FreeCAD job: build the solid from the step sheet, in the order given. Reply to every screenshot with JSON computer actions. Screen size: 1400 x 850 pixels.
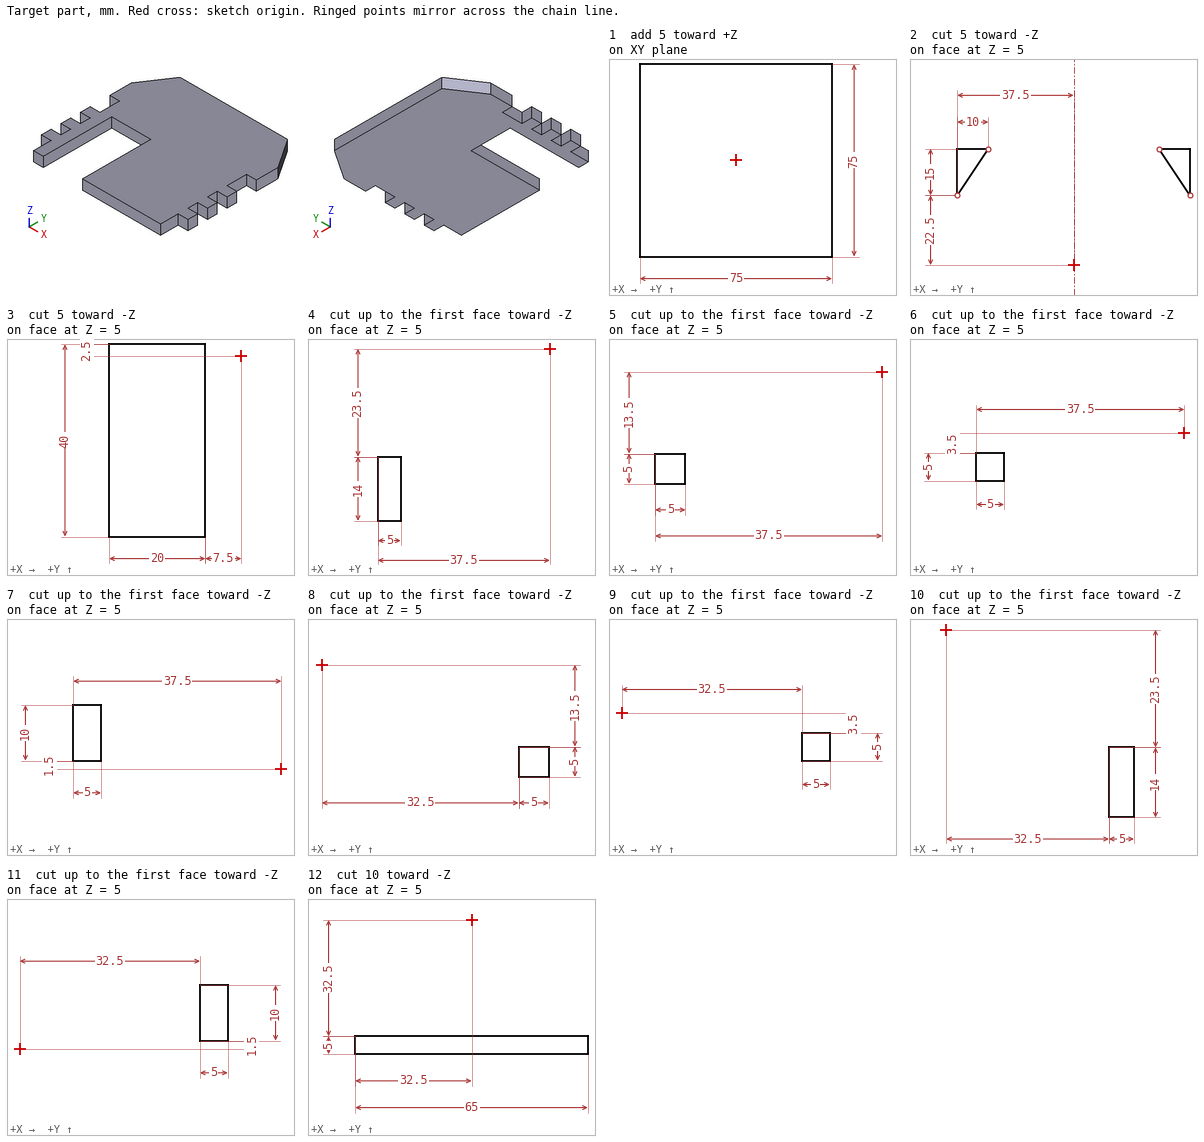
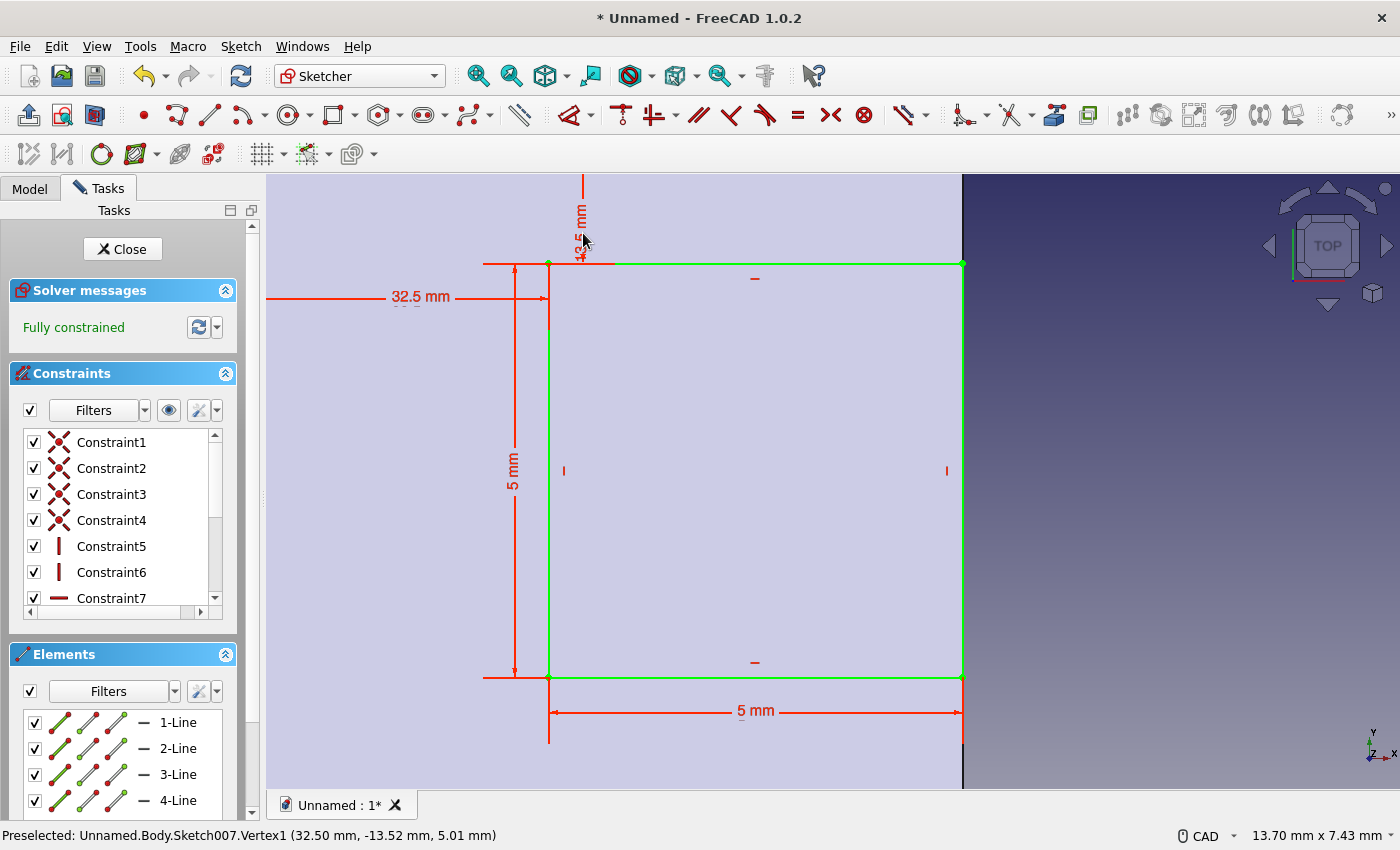
{"action": "left_click", "coordinate": [123, 249]}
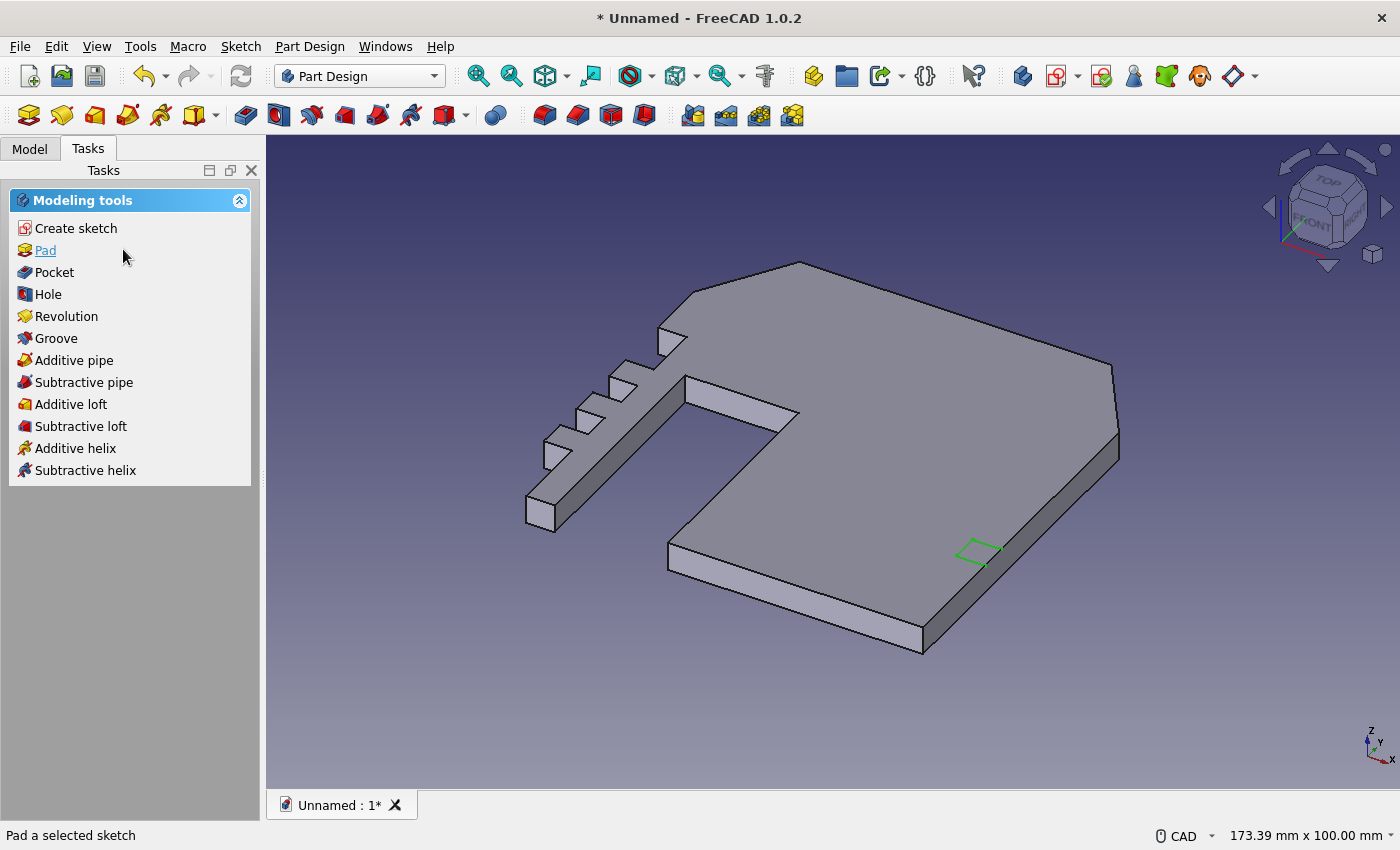
{"action": "left_click", "coordinate": [246, 116]}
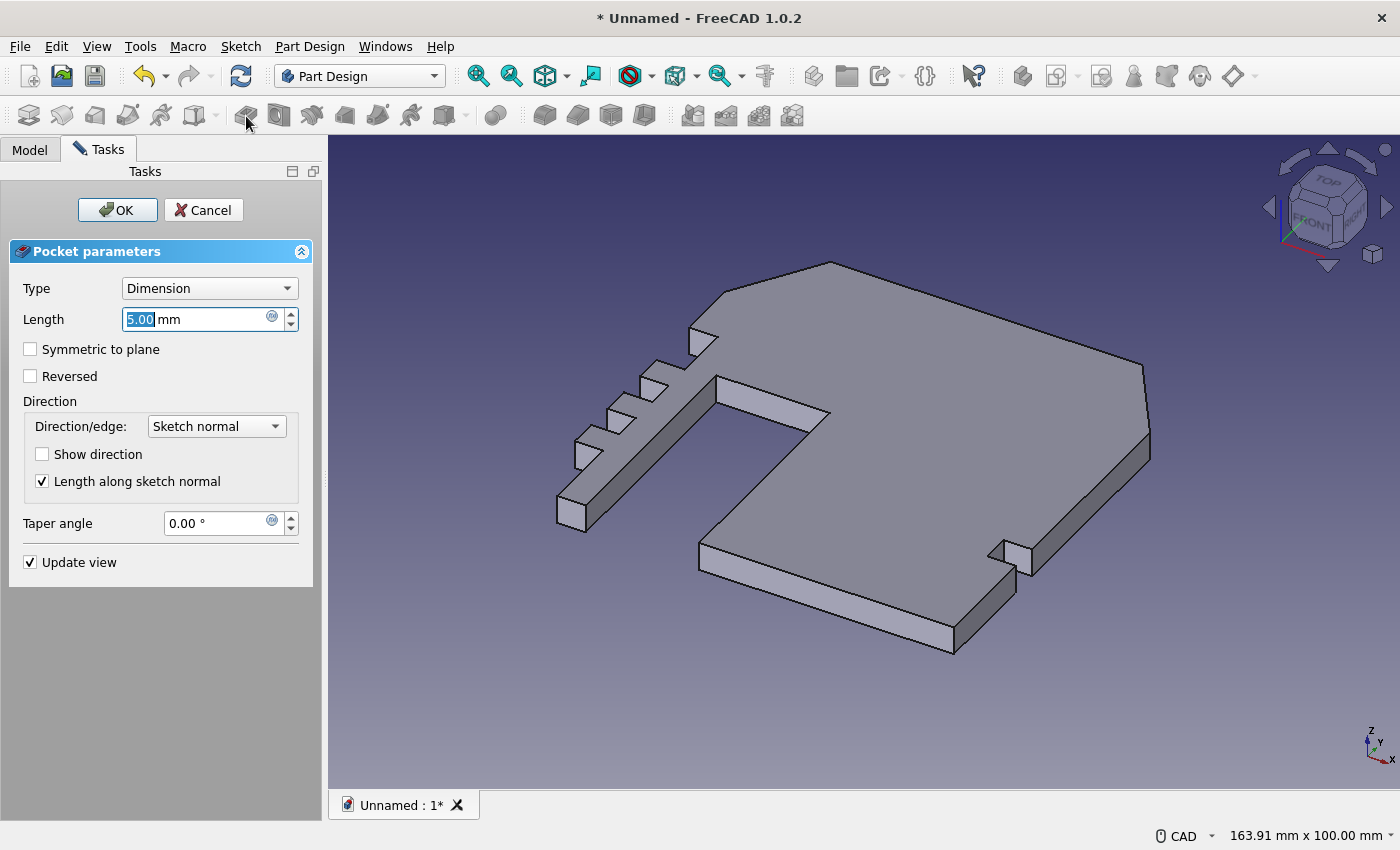
{"action": "left_click", "coordinate": [210, 288]}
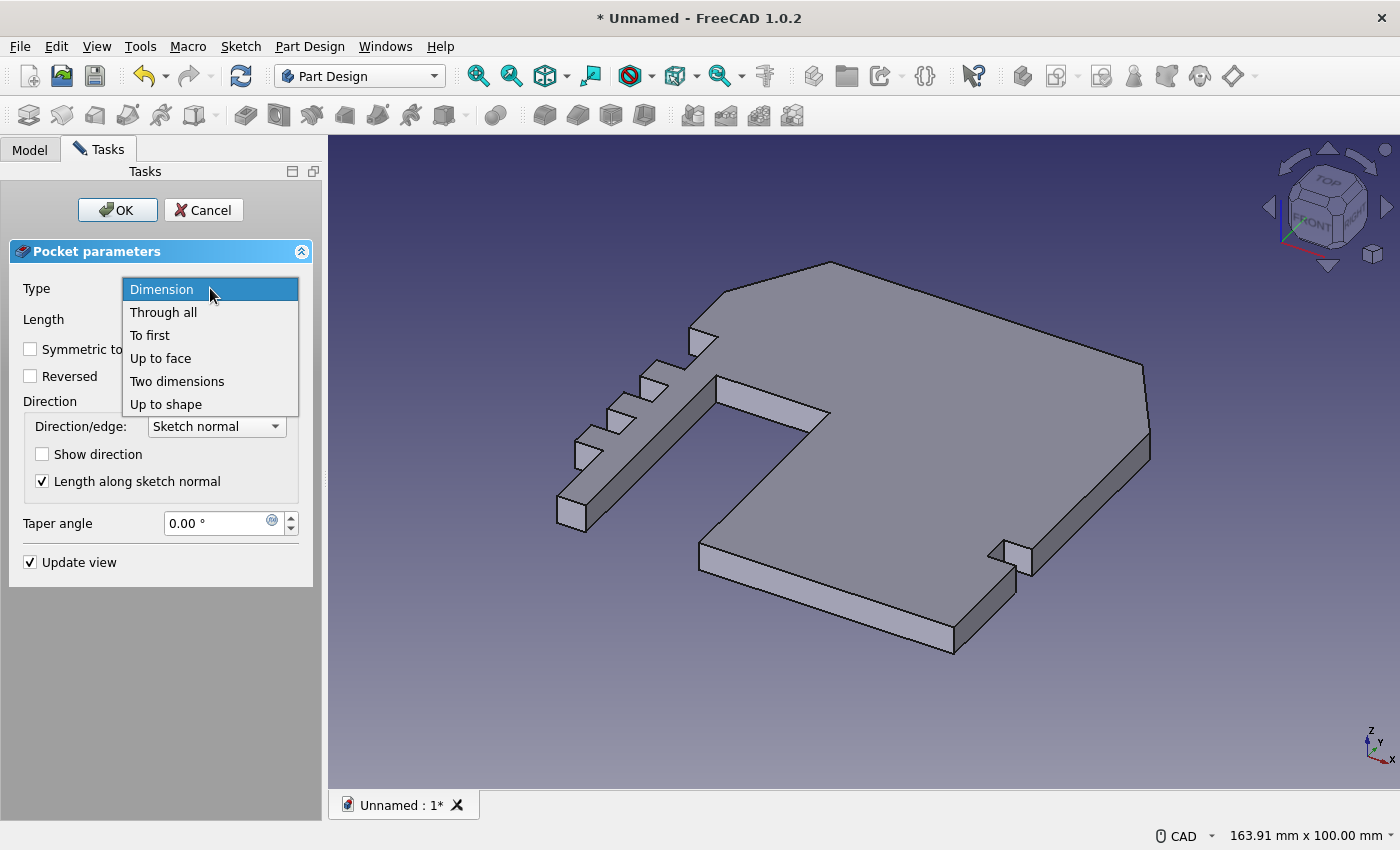
{"action": "left_click", "coordinate": [208, 336]}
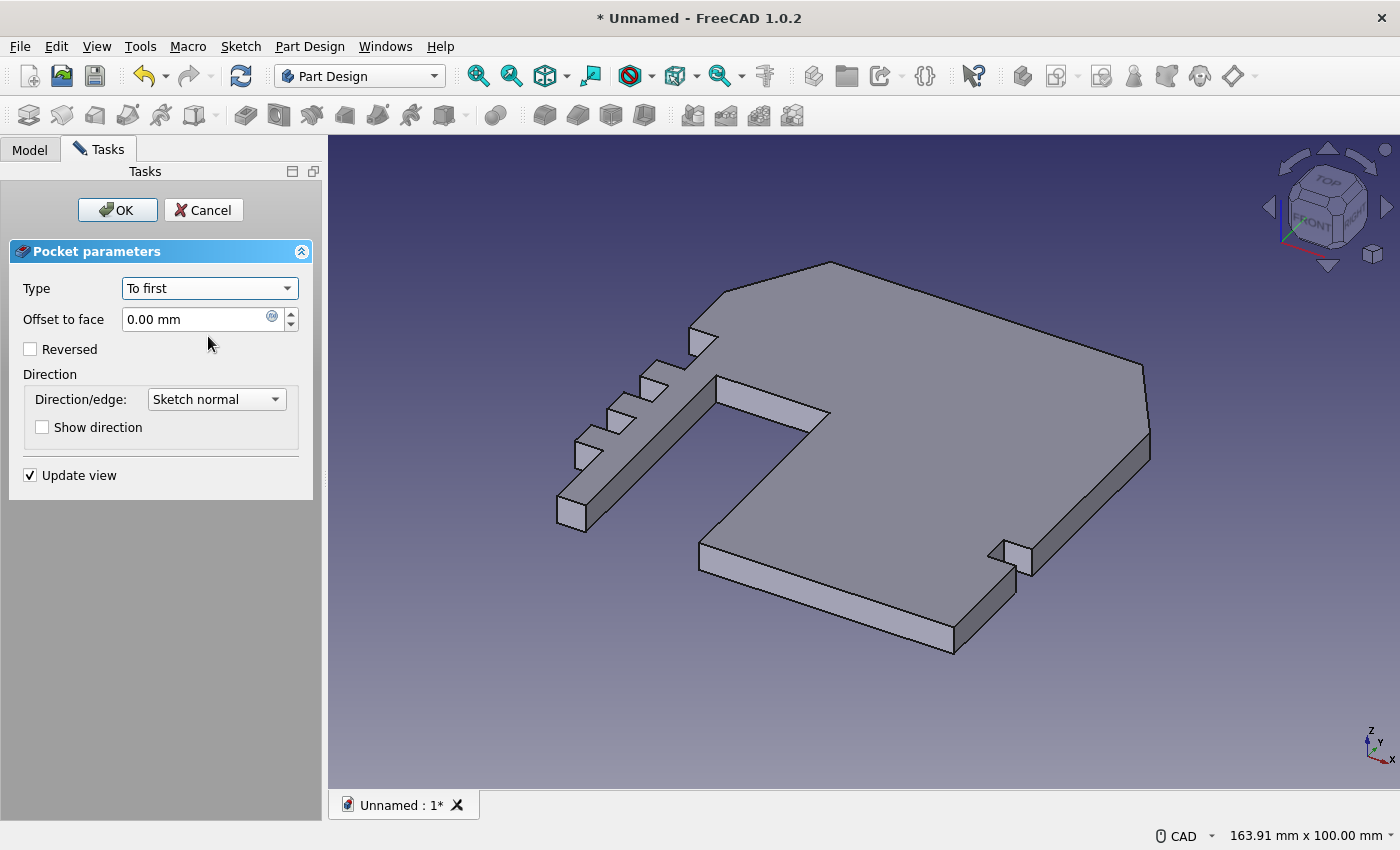
{"action": "left_click", "coordinate": [118, 210]}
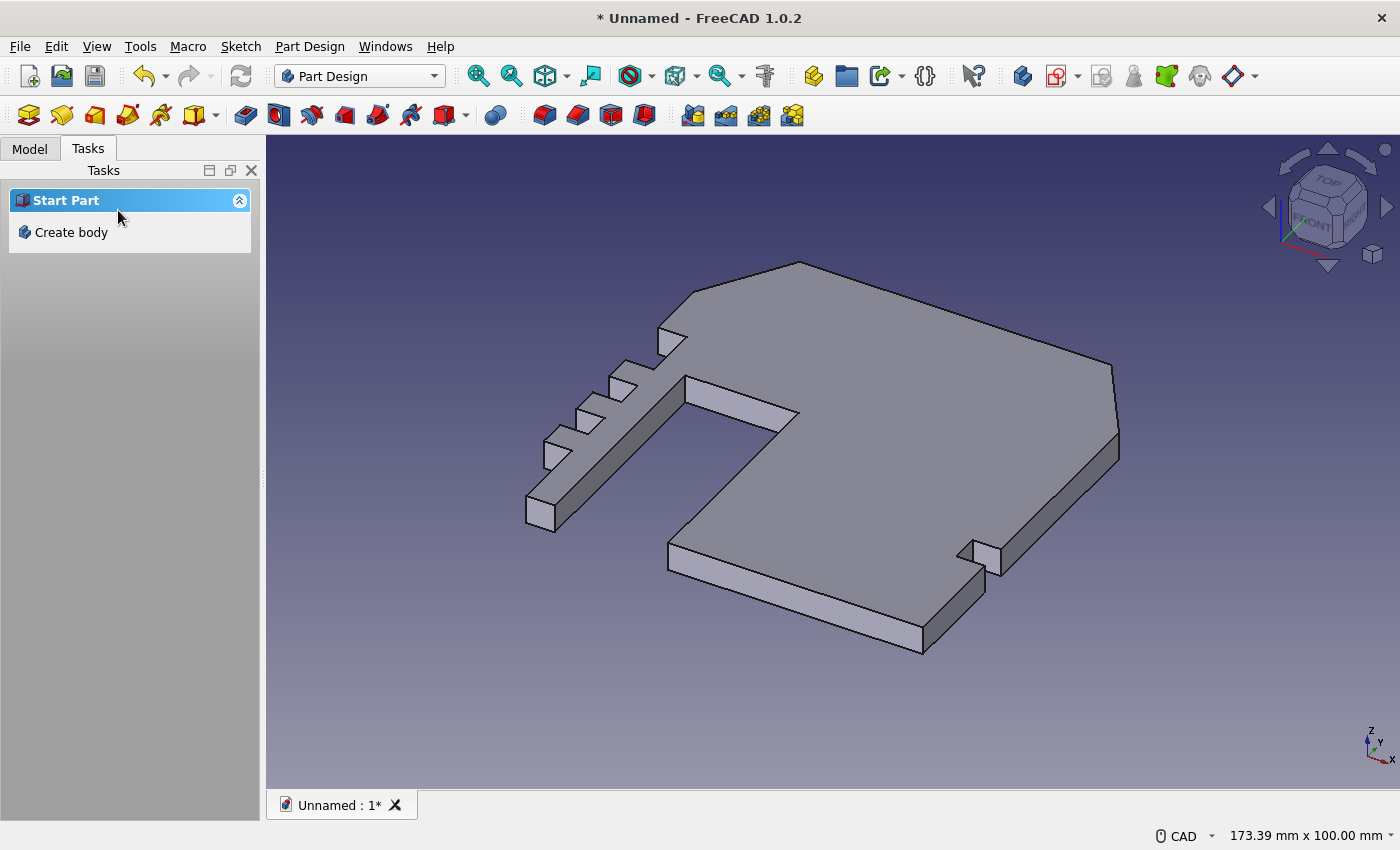
{"action": "left_click", "coordinate": [929, 420]}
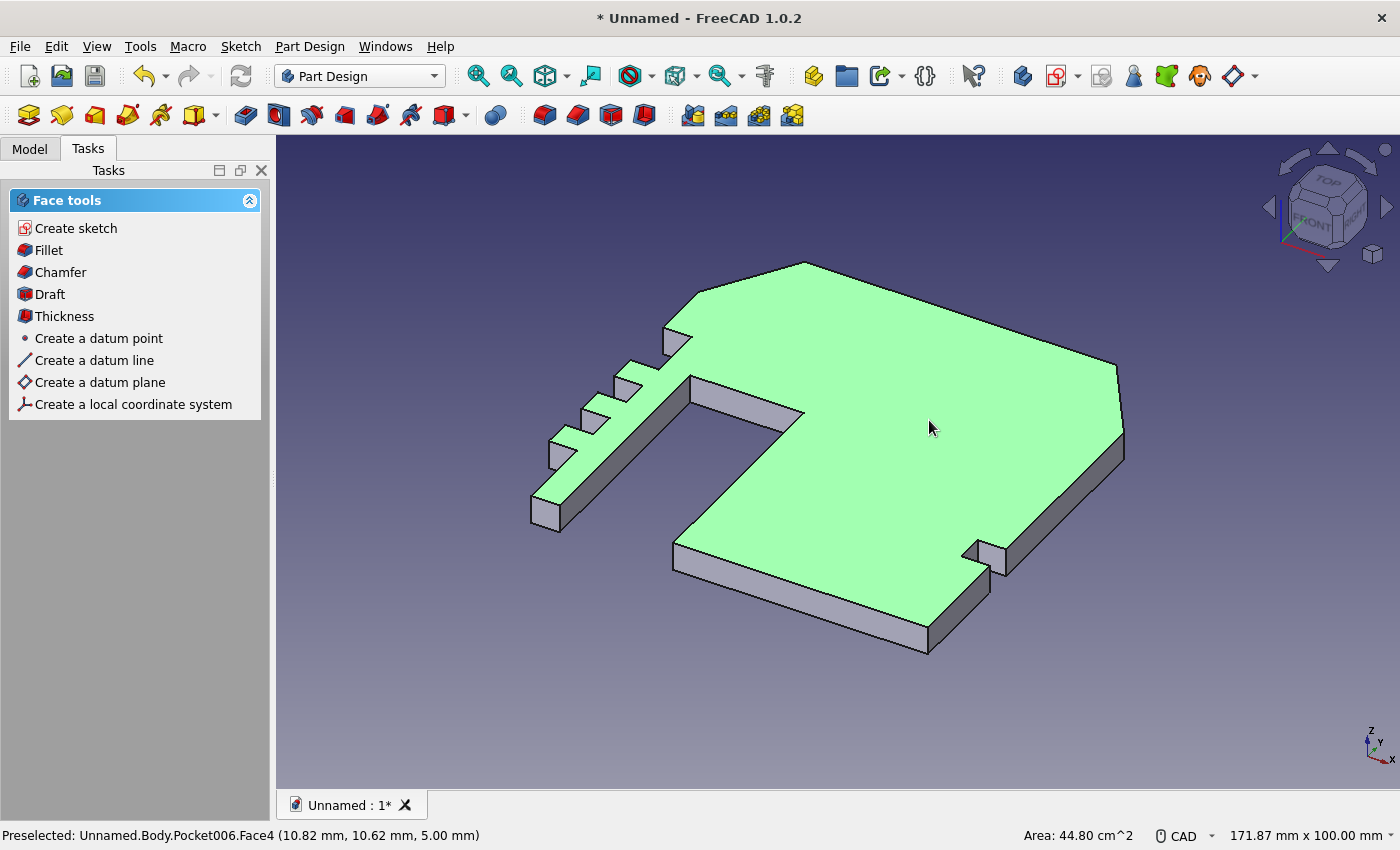
{"action": "left_click", "coordinate": [1056, 76]}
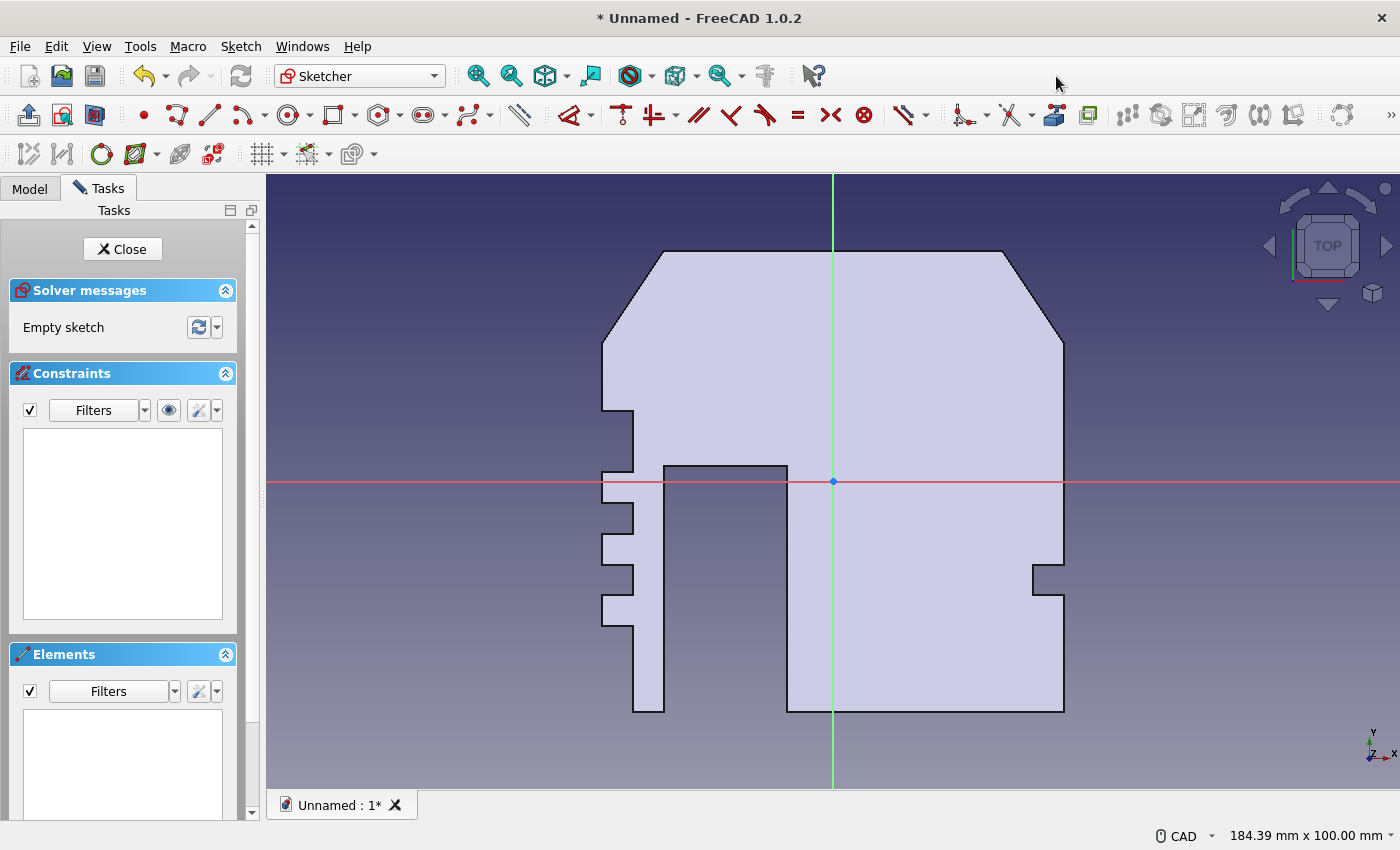
{"action": "scroll", "coordinate": [1071, 521], "scroll_direction": "up", "scroll_amount": 13}